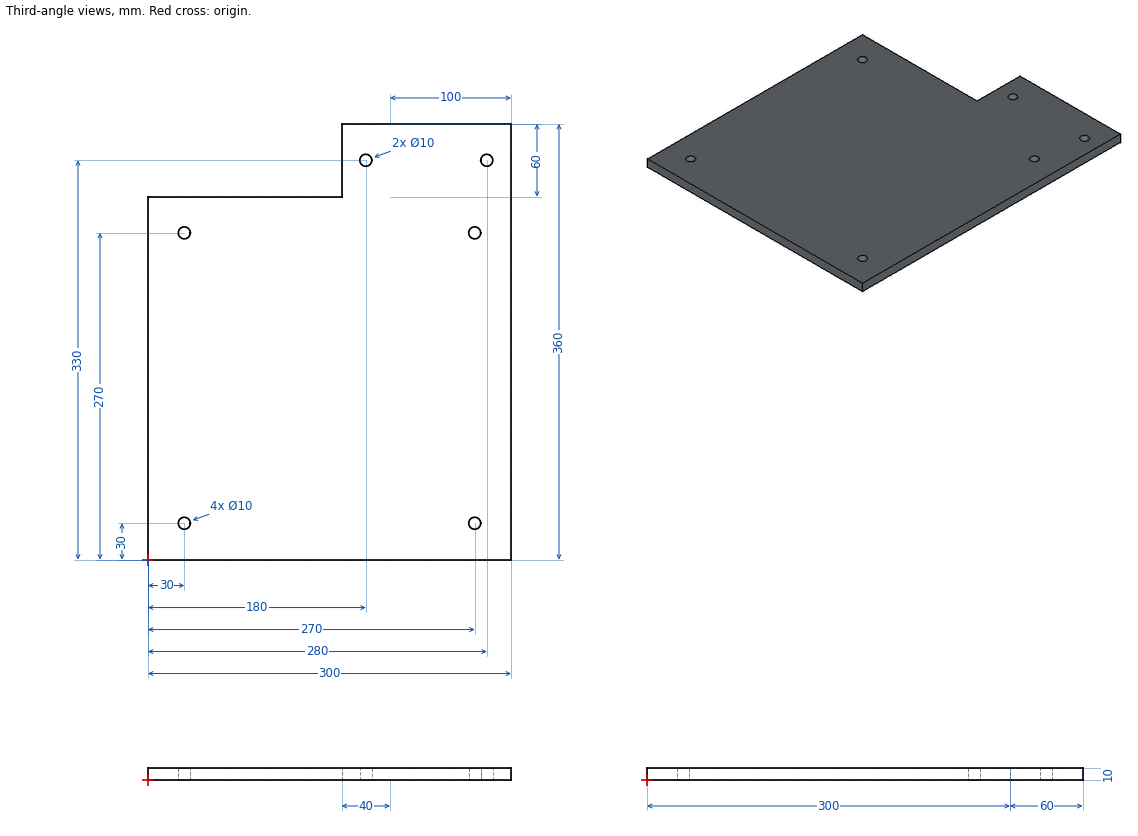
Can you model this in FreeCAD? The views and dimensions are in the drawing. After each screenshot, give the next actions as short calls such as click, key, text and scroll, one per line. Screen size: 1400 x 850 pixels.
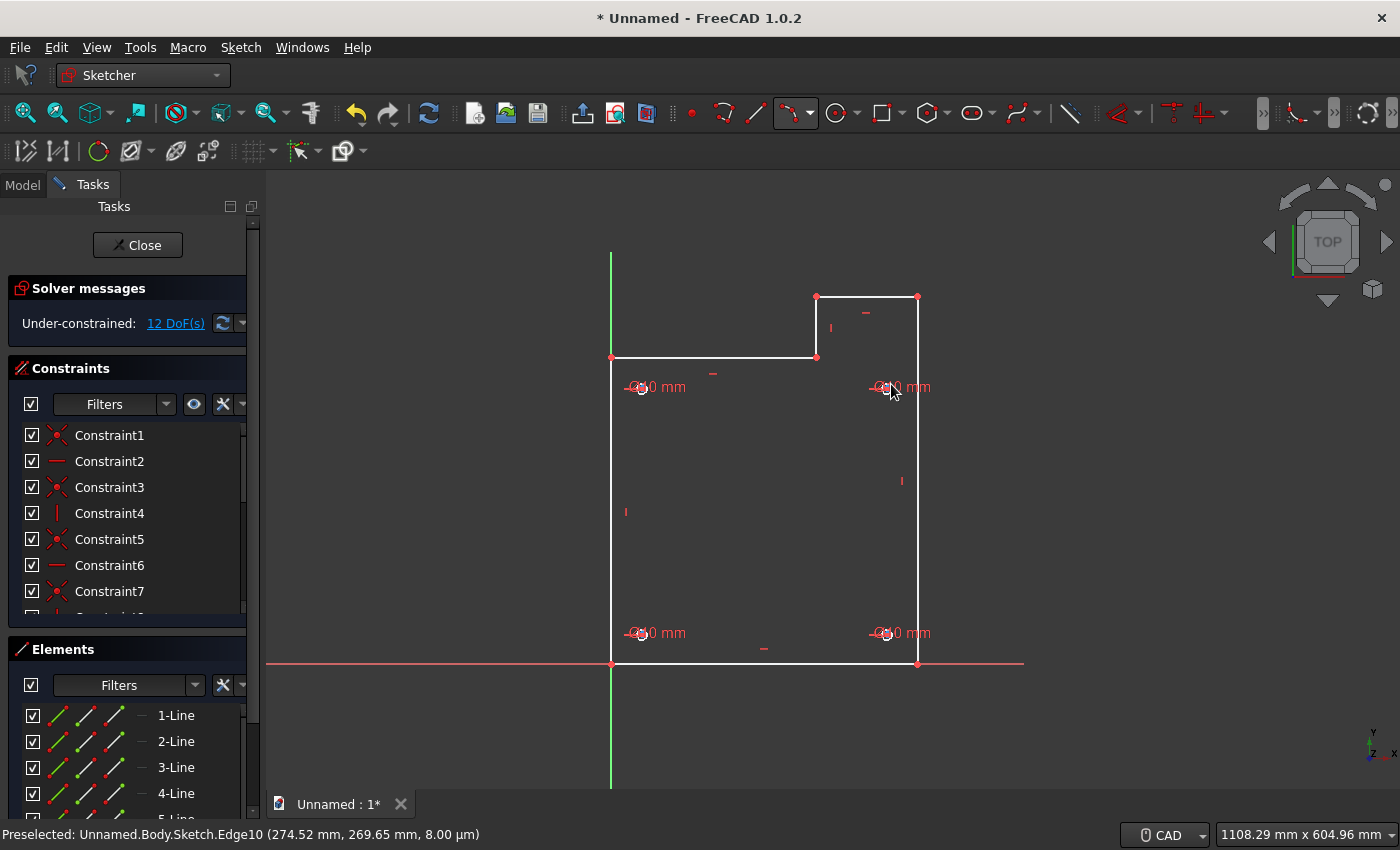
click(642, 635)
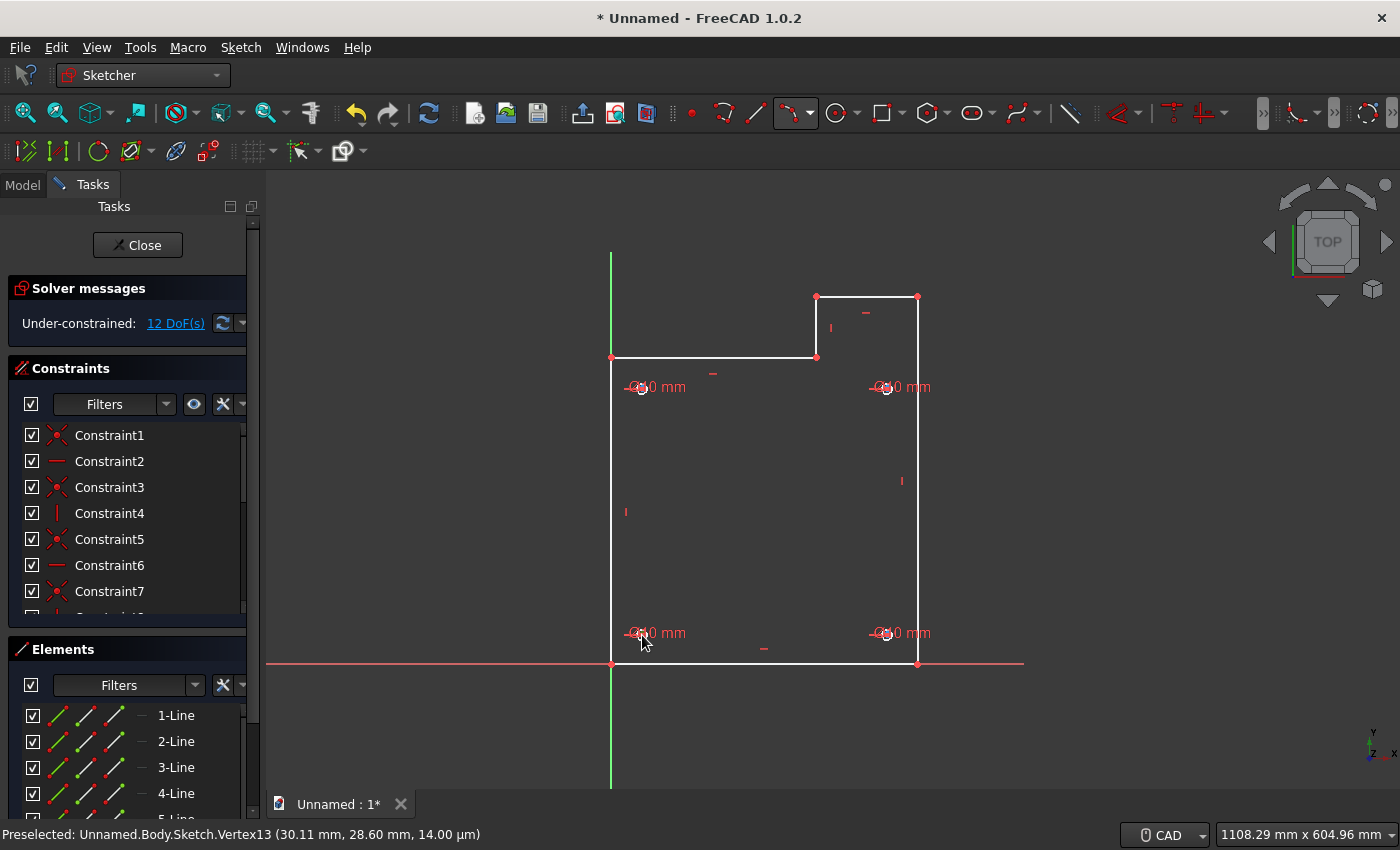
click(887, 635)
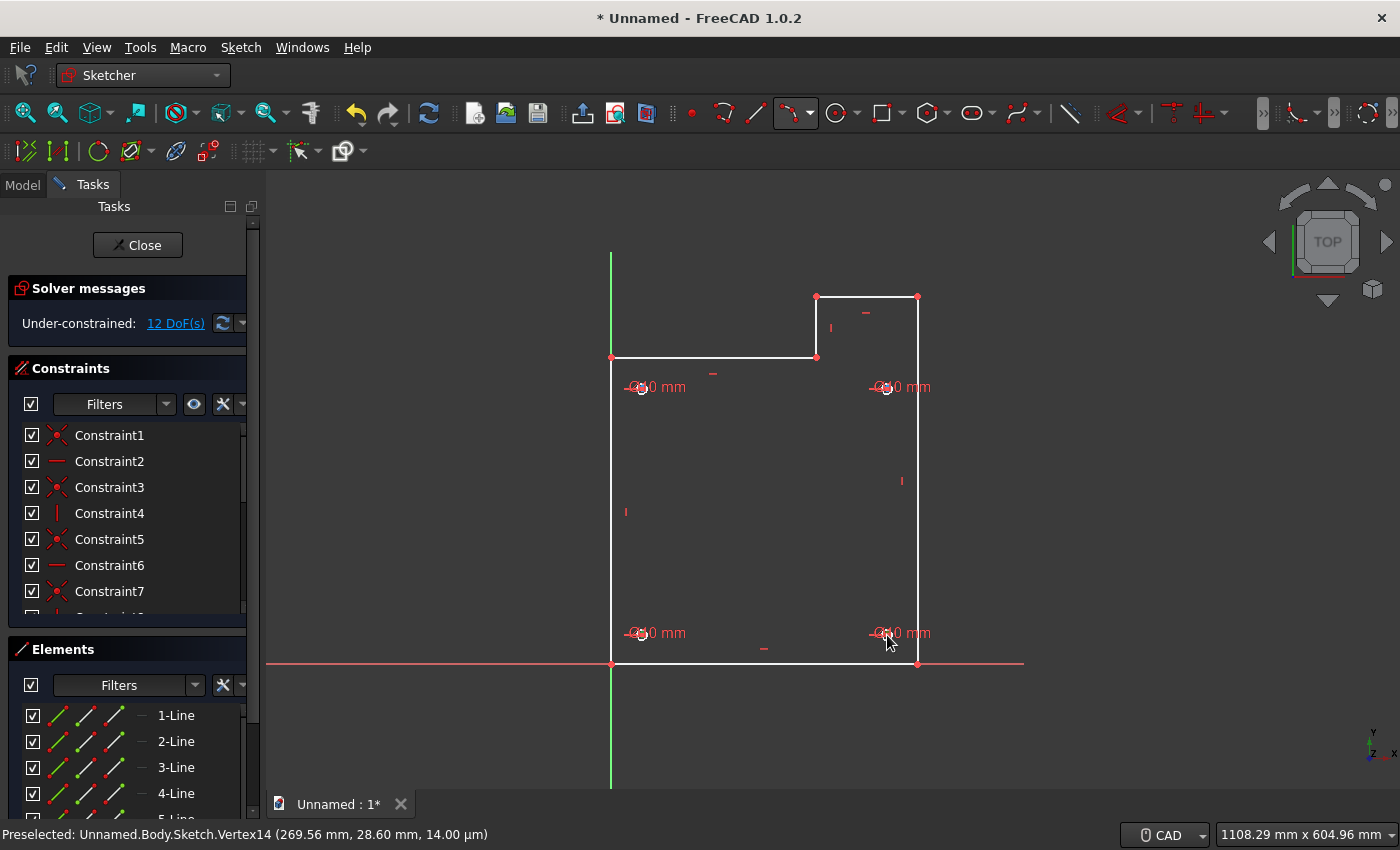
click(1226, 114)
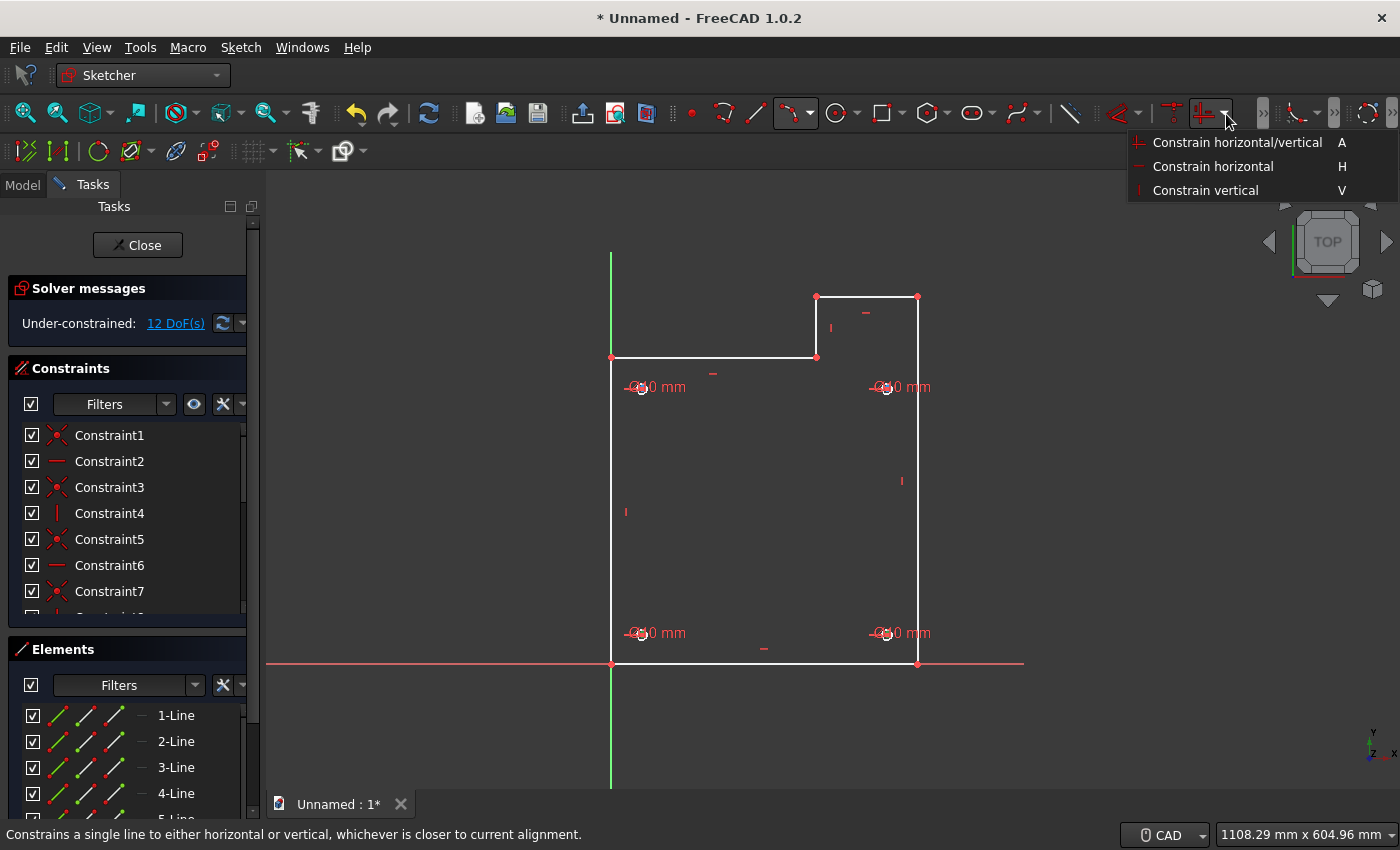
click(1263, 166)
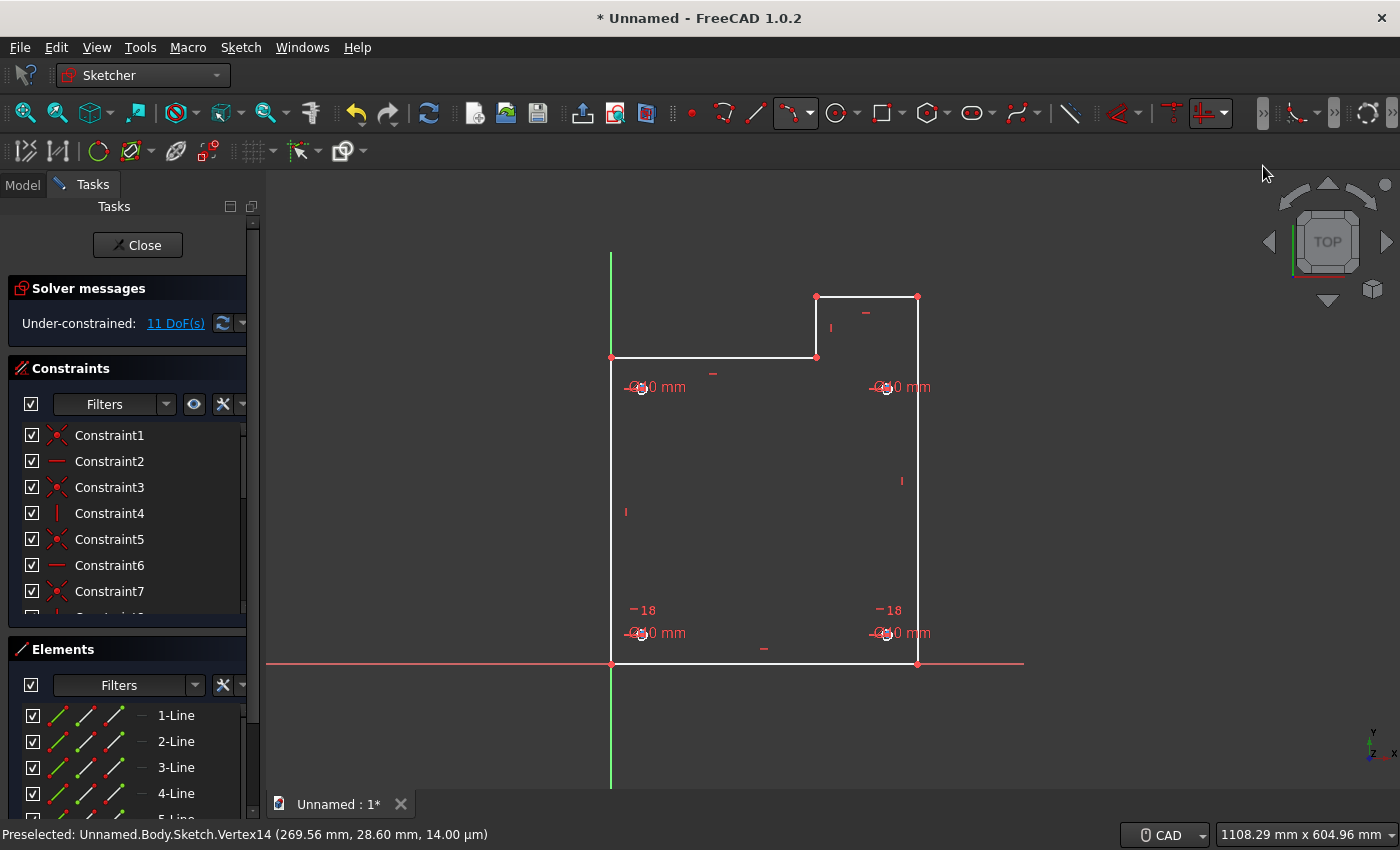
click(1118, 114)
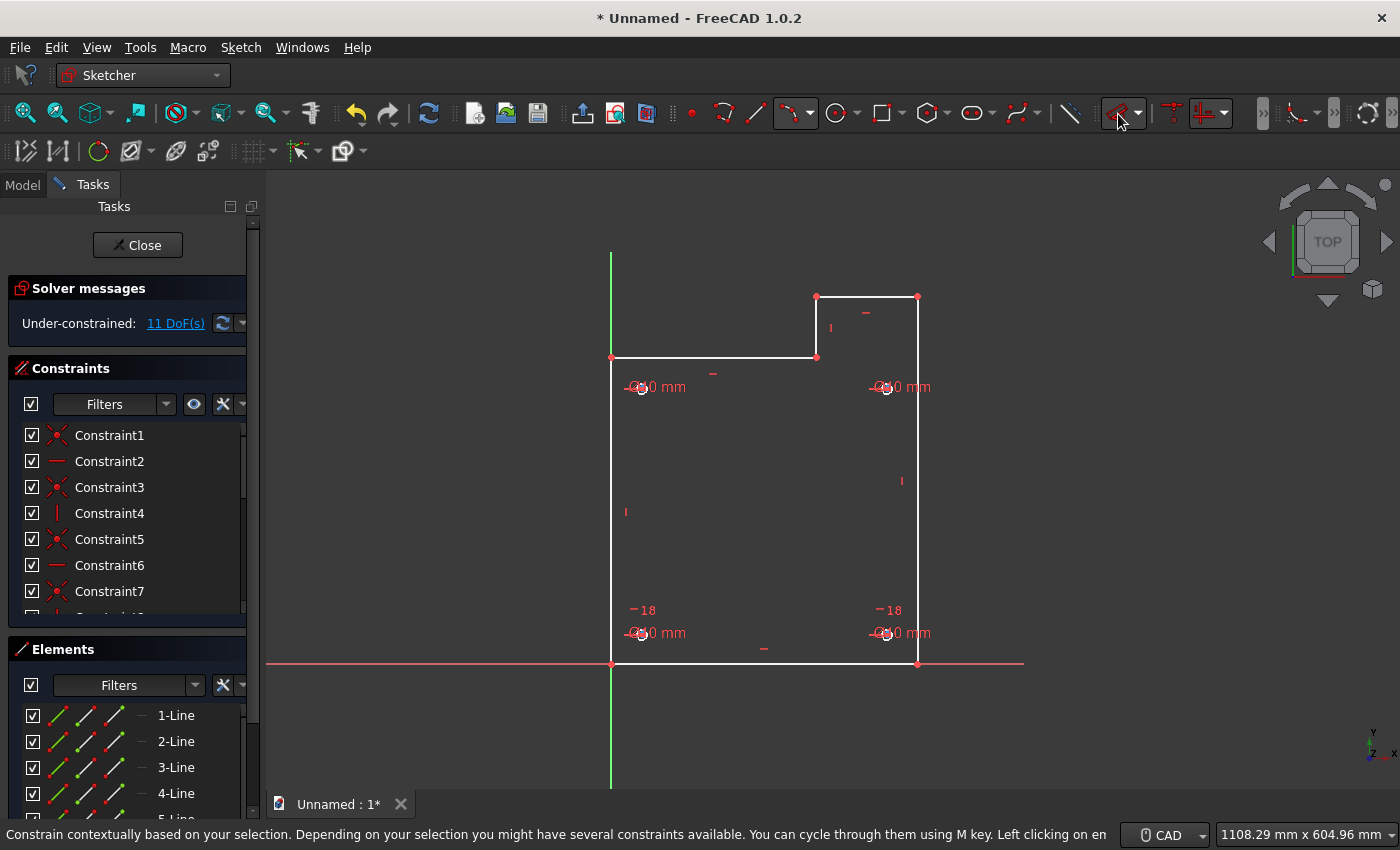
click(816, 315)
click(850, 327)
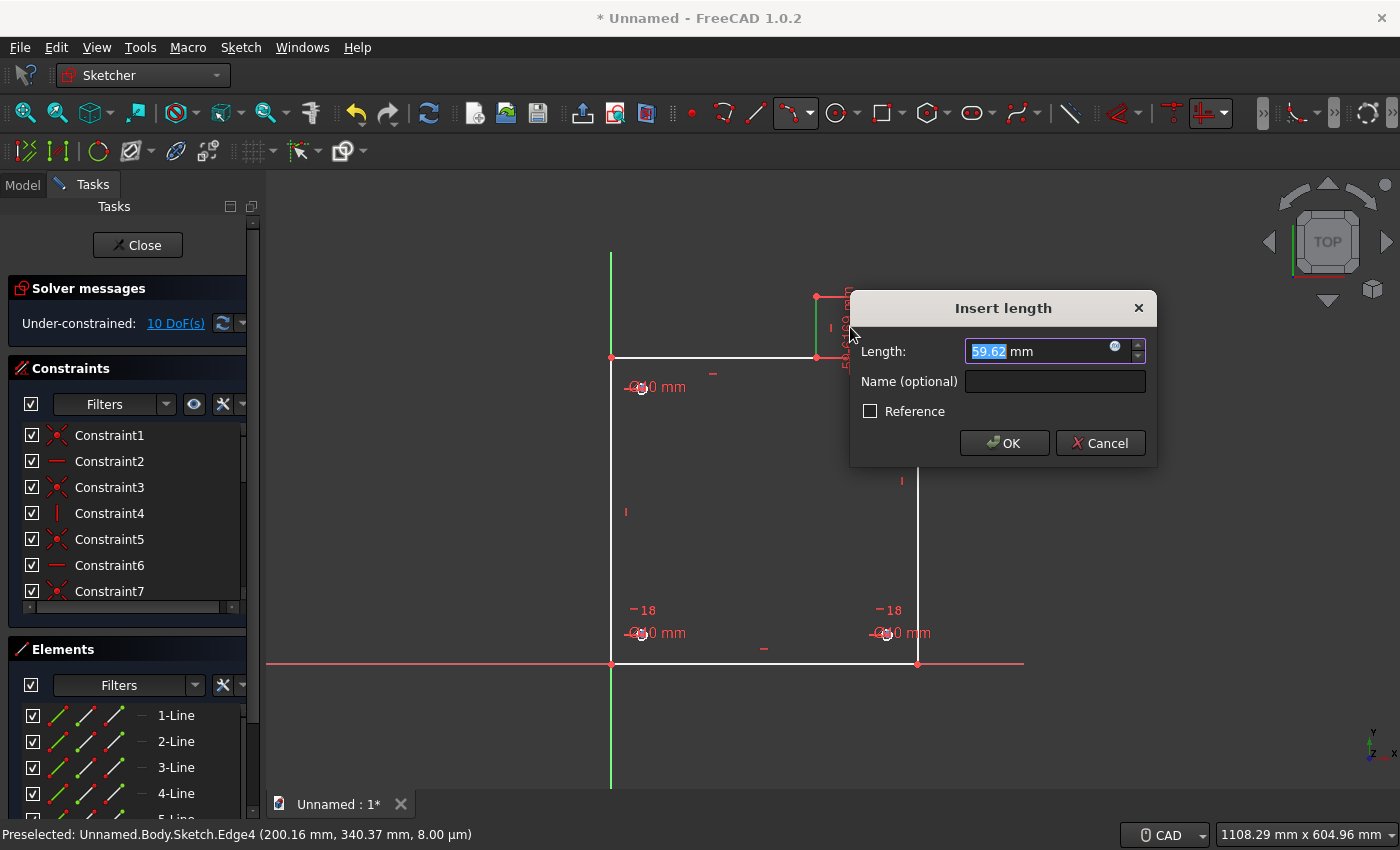
text(60)
key(Return)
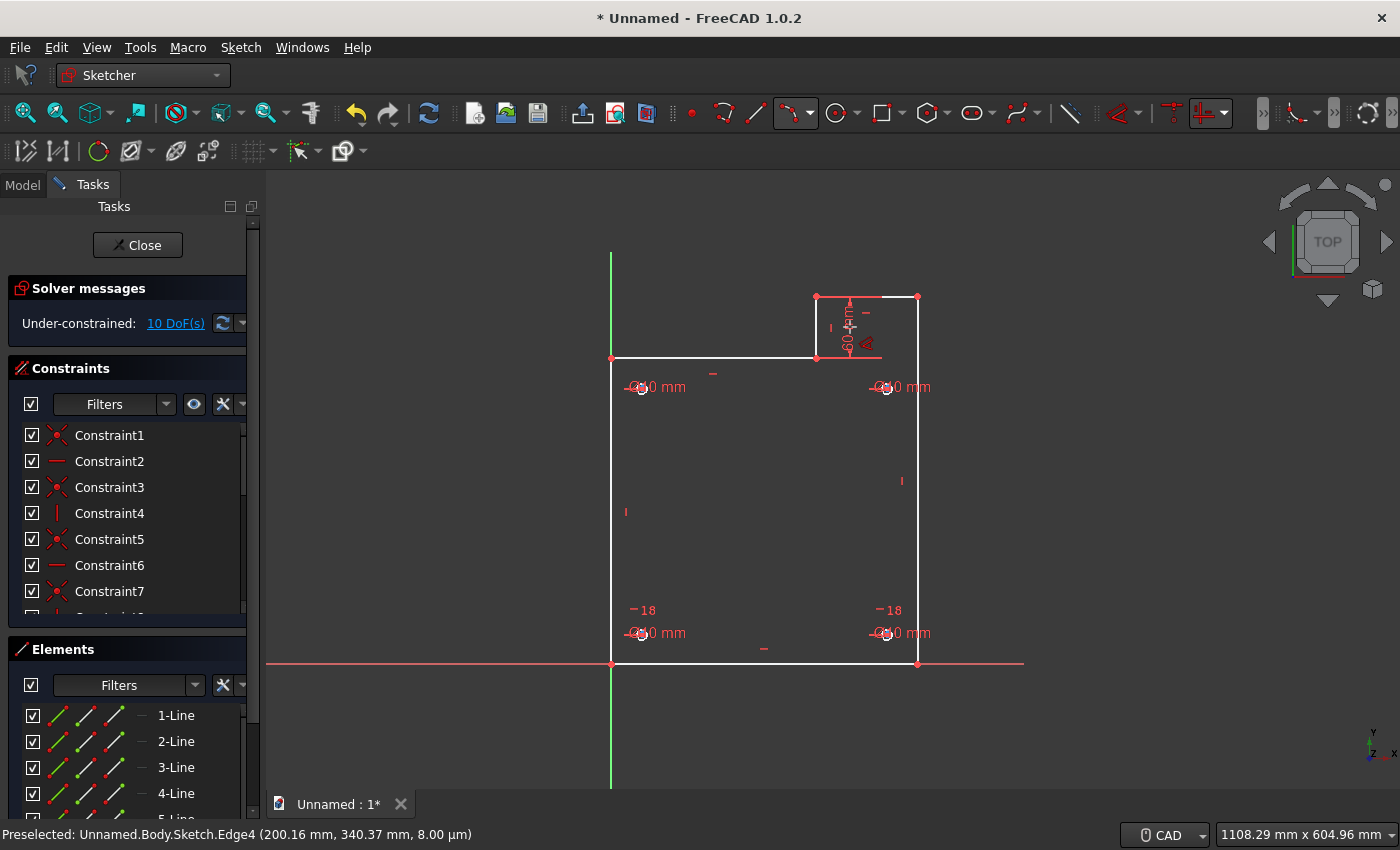
scroll(642, 635, up, 2)